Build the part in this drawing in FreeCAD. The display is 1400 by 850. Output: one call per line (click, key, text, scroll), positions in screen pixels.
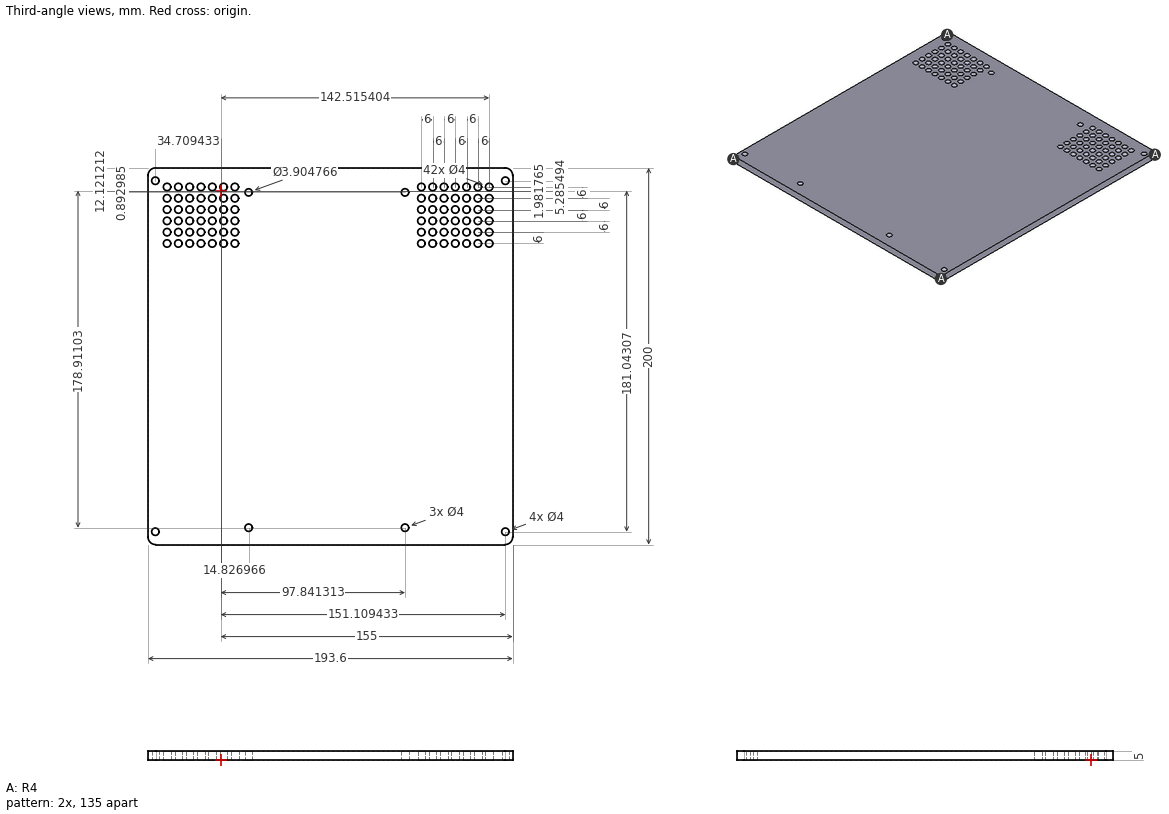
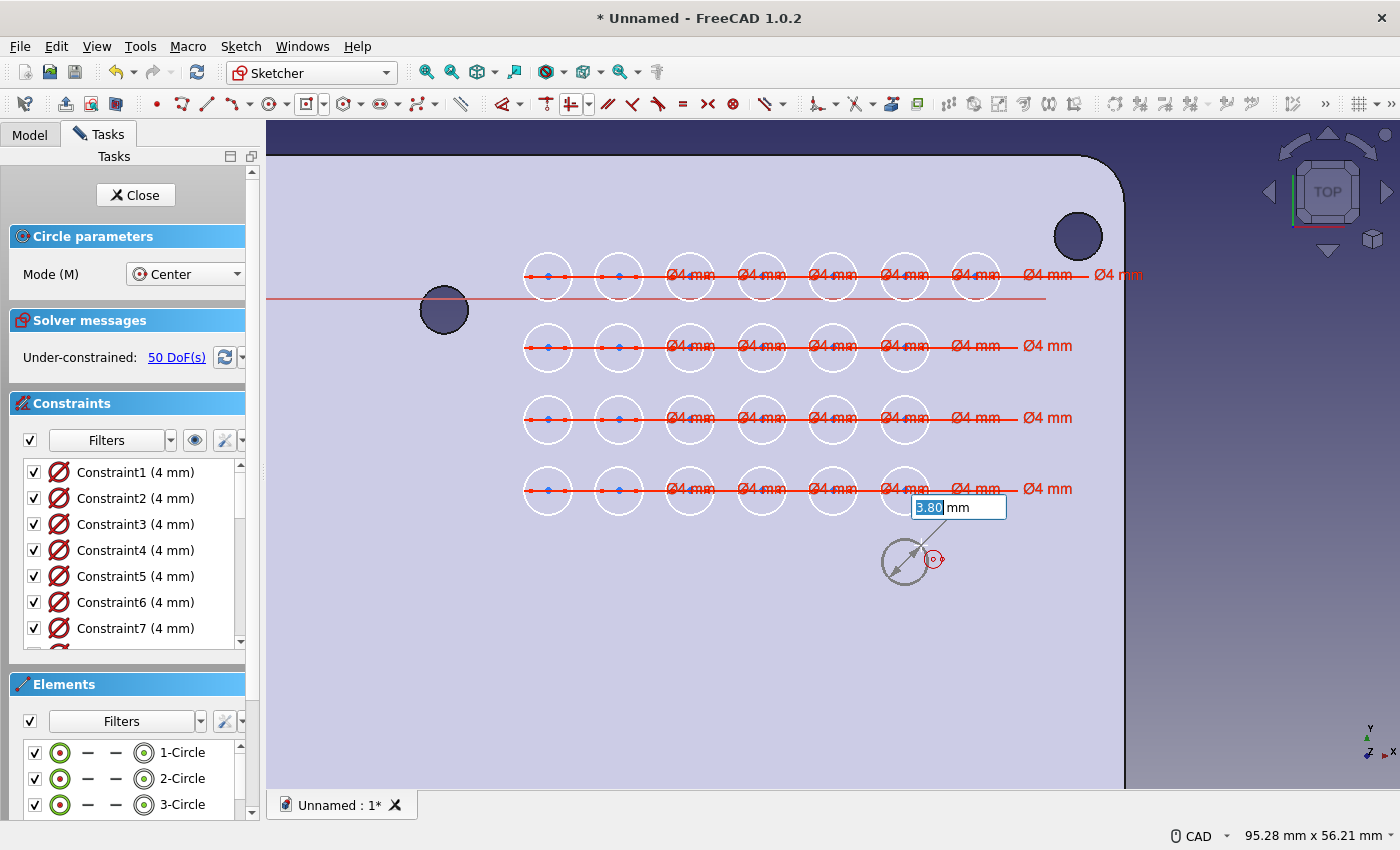
text(4)
key(Return)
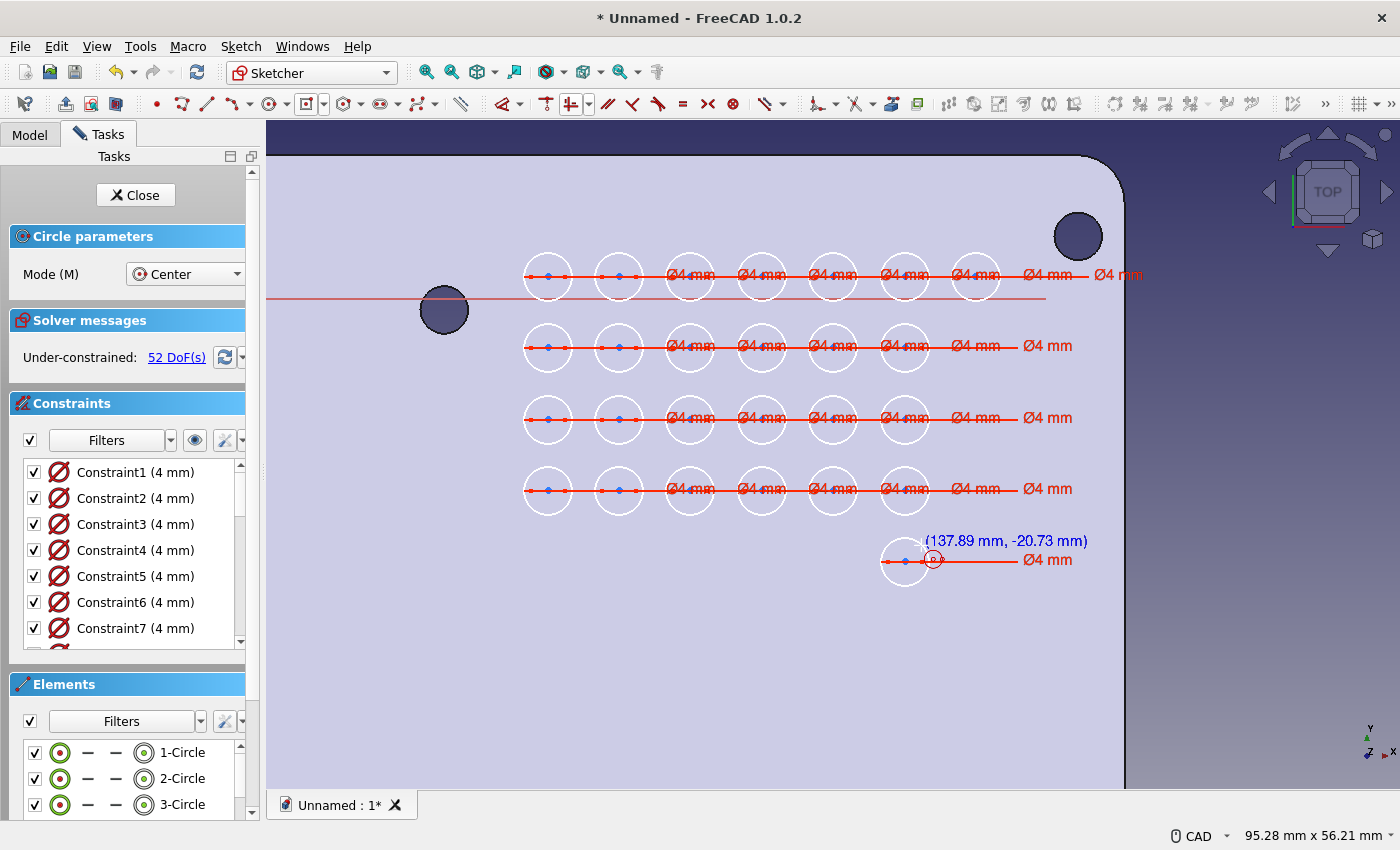
click(833, 561)
move(850, 545)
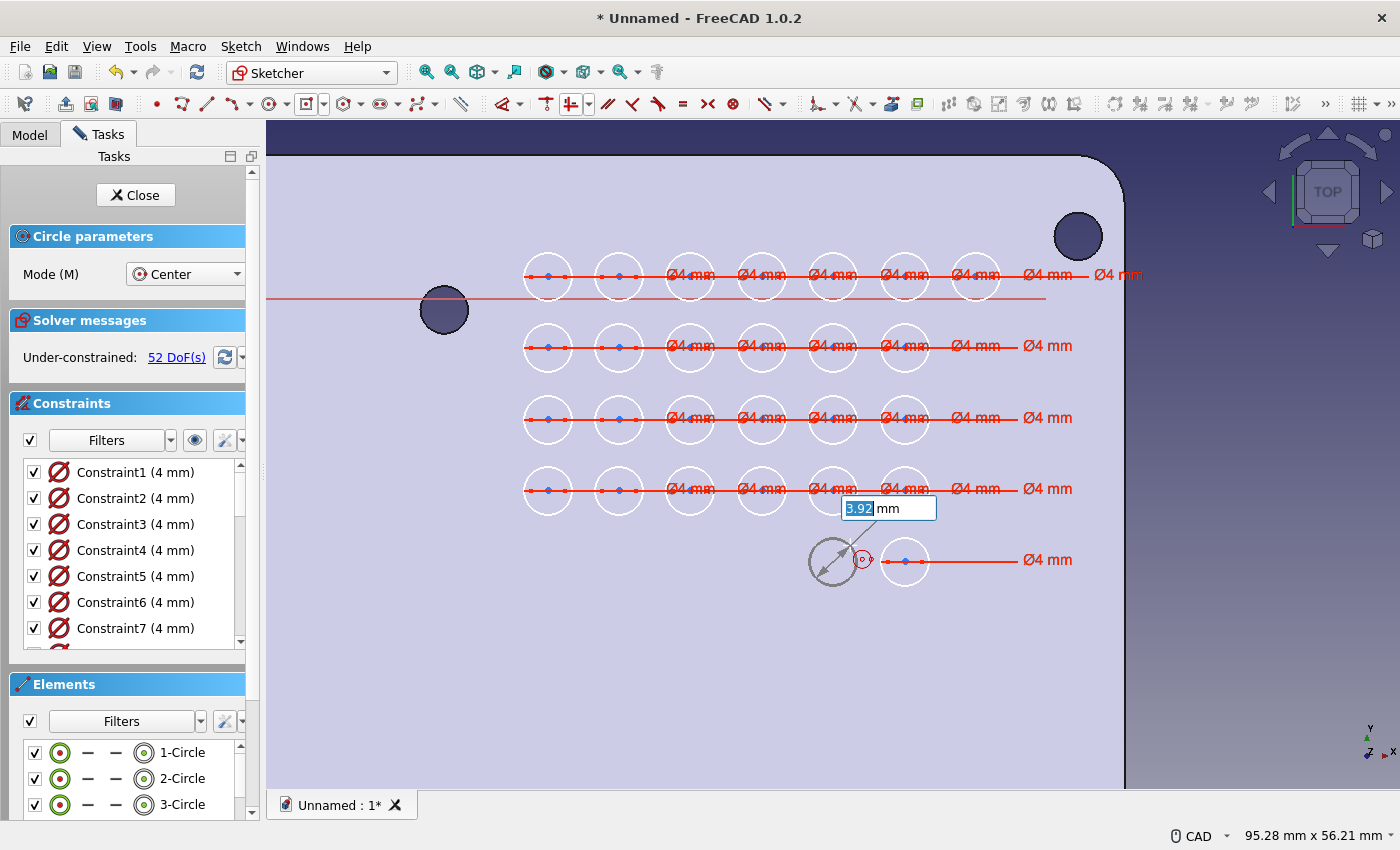
text(4)
key(Return)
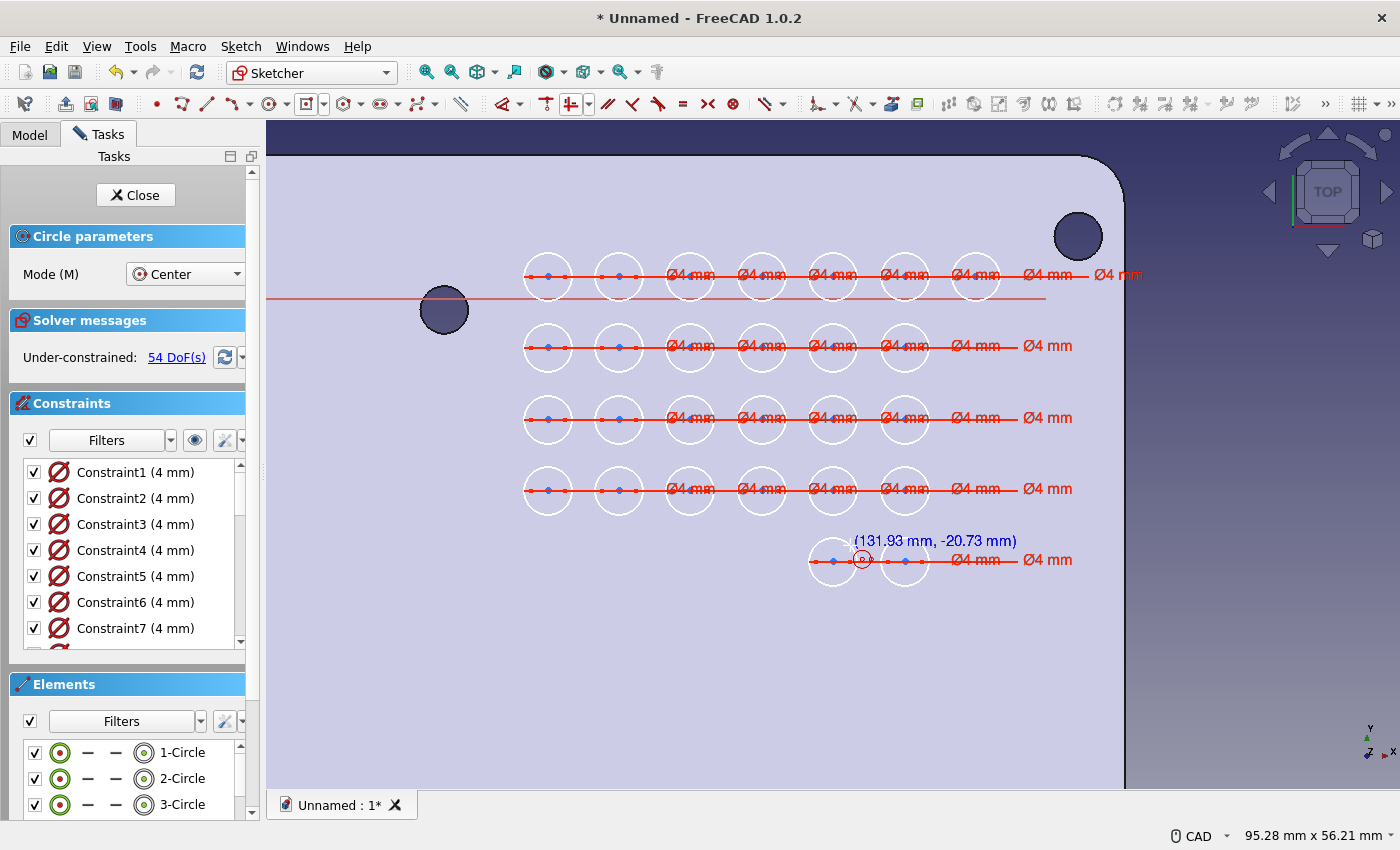
click(762, 561)
move(779, 545)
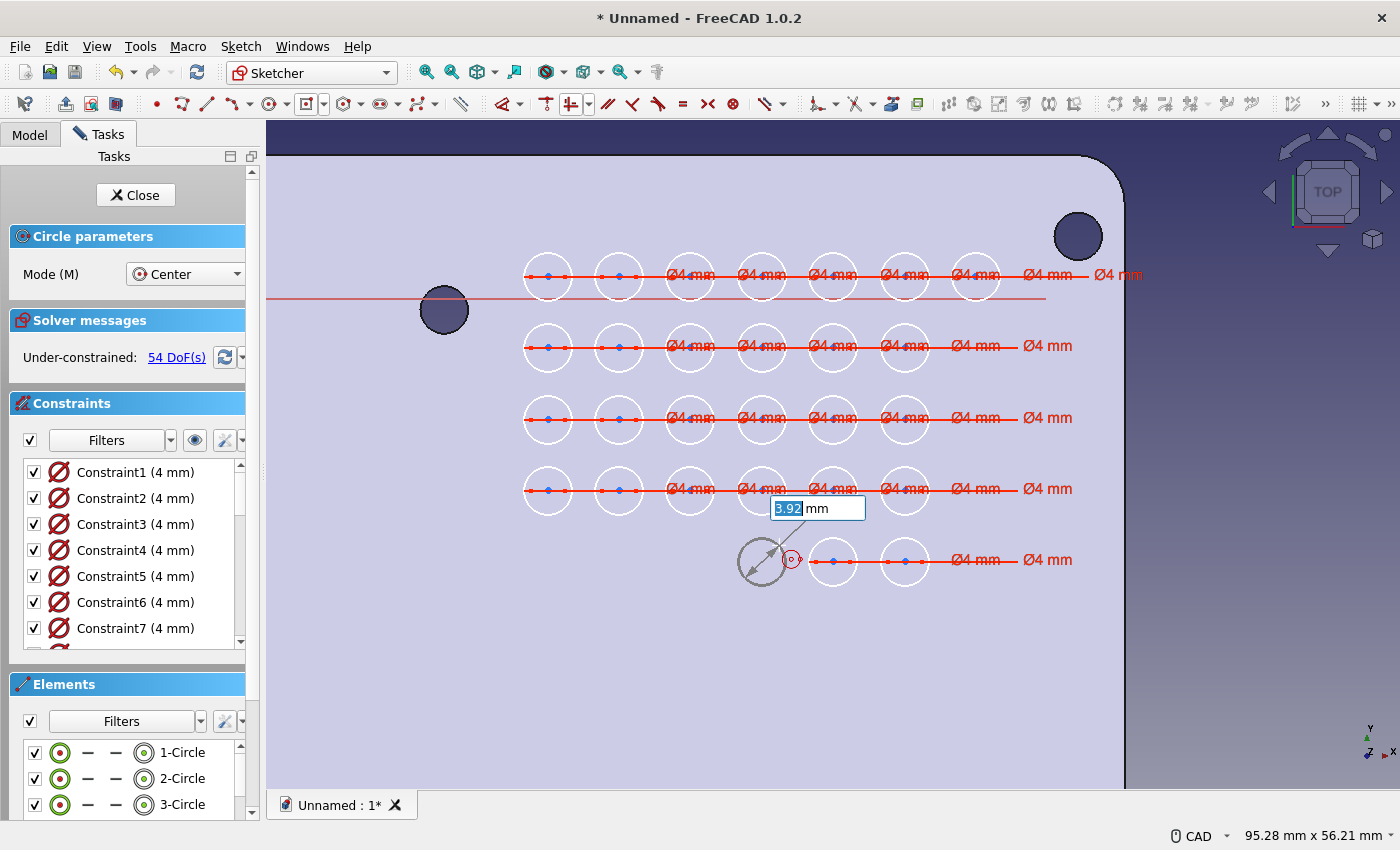
text(4)
key(Return)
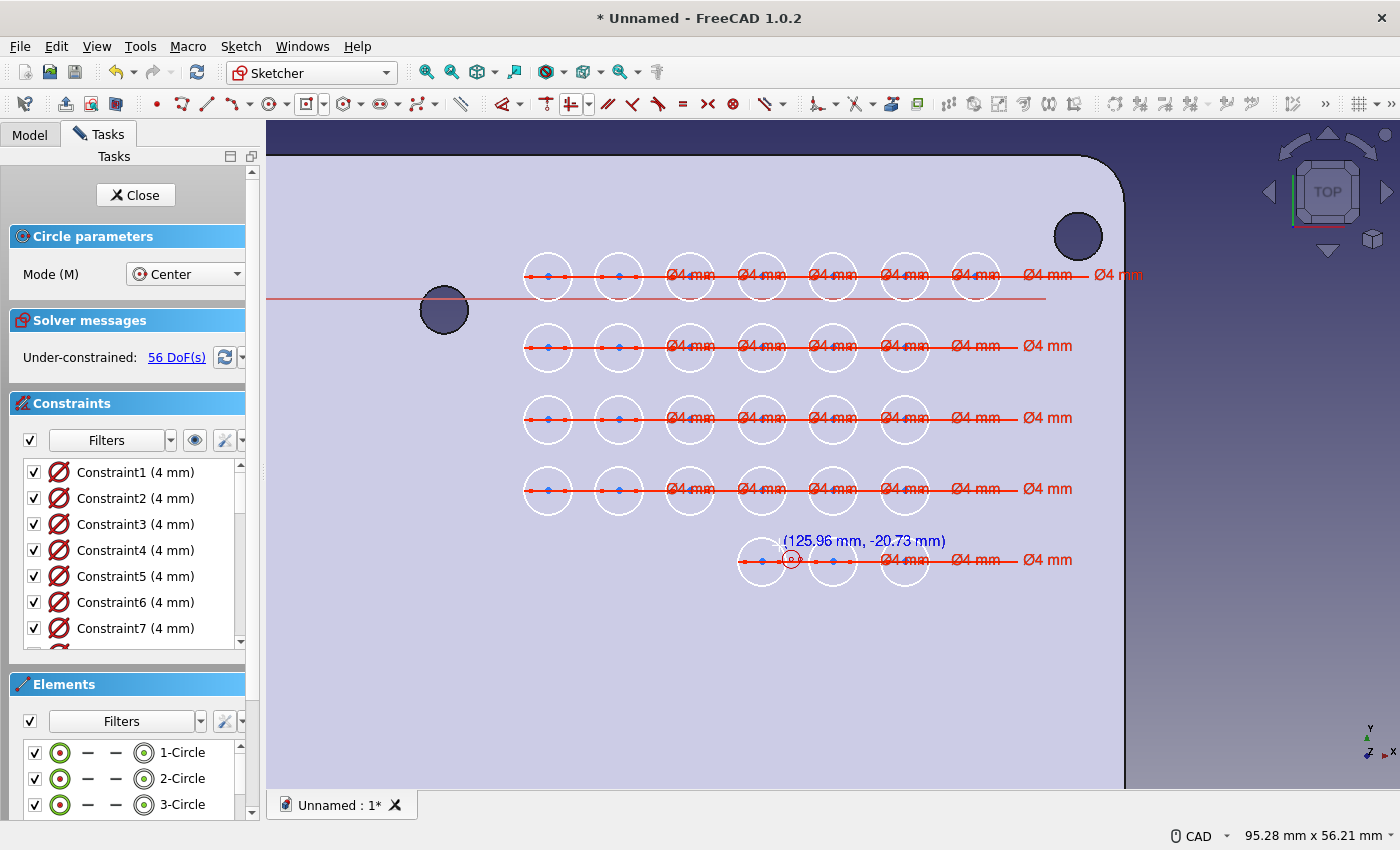
click(690, 561)
move(707, 545)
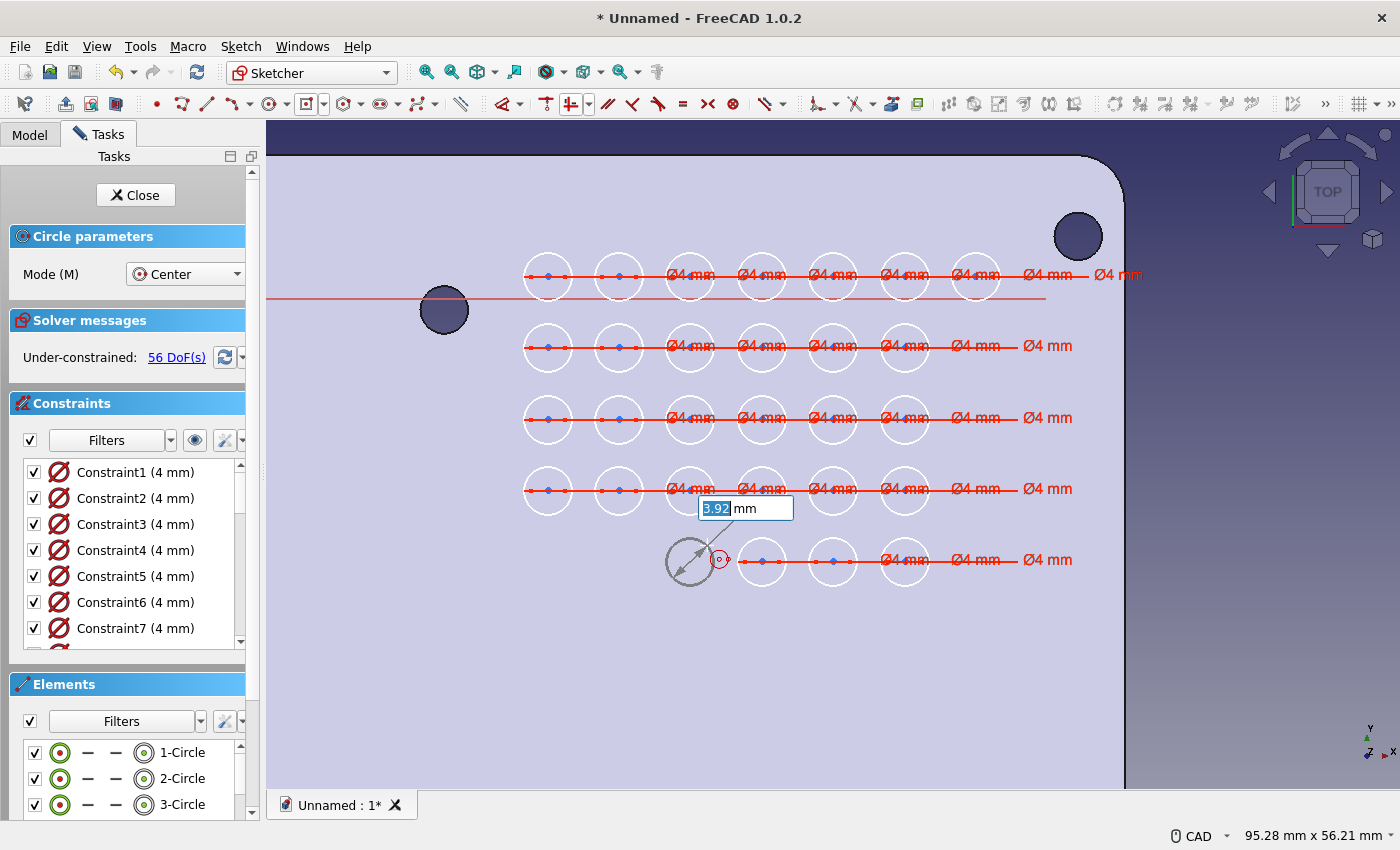
text(4)
key(Return)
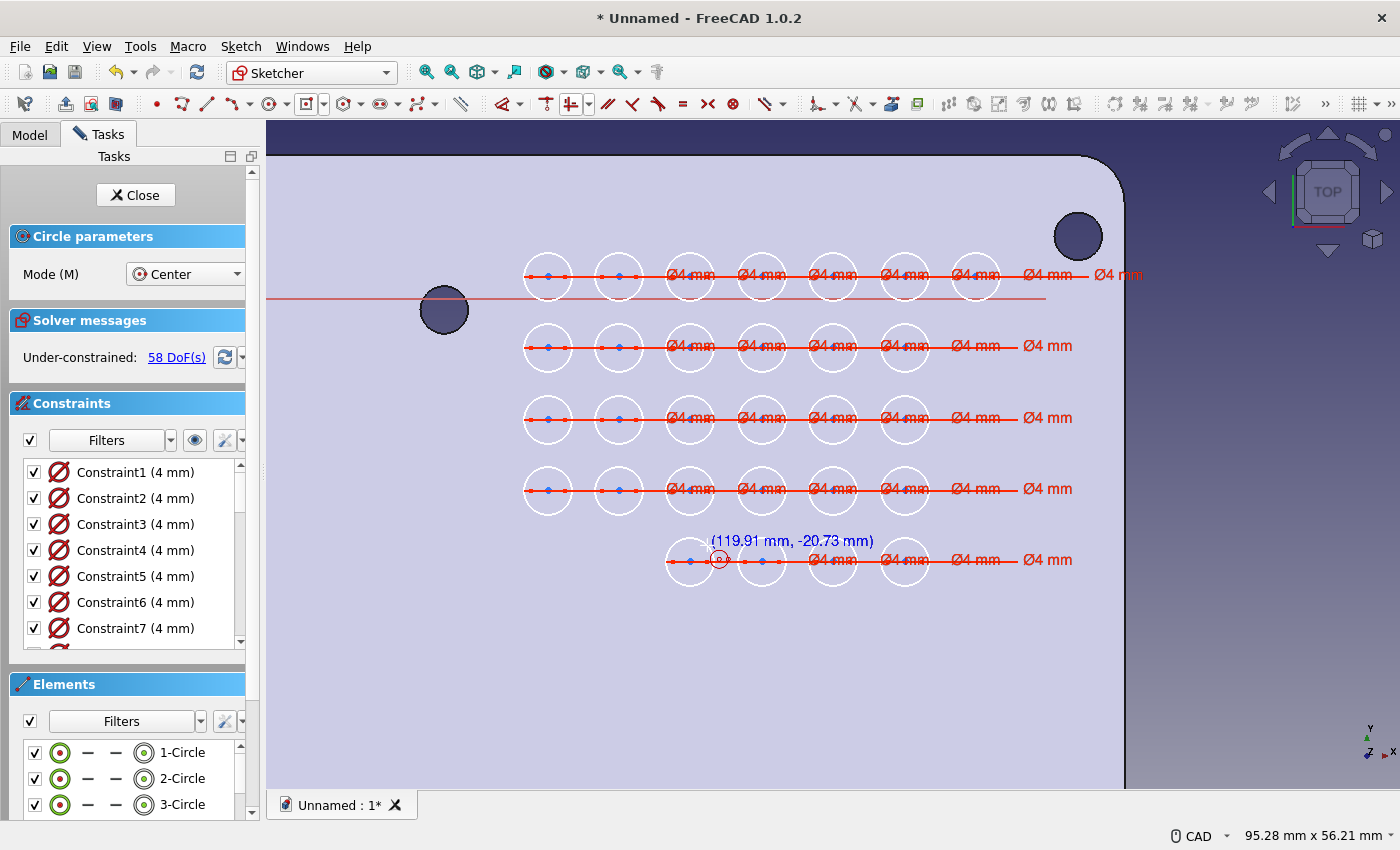
click(619, 561)
move(636, 545)